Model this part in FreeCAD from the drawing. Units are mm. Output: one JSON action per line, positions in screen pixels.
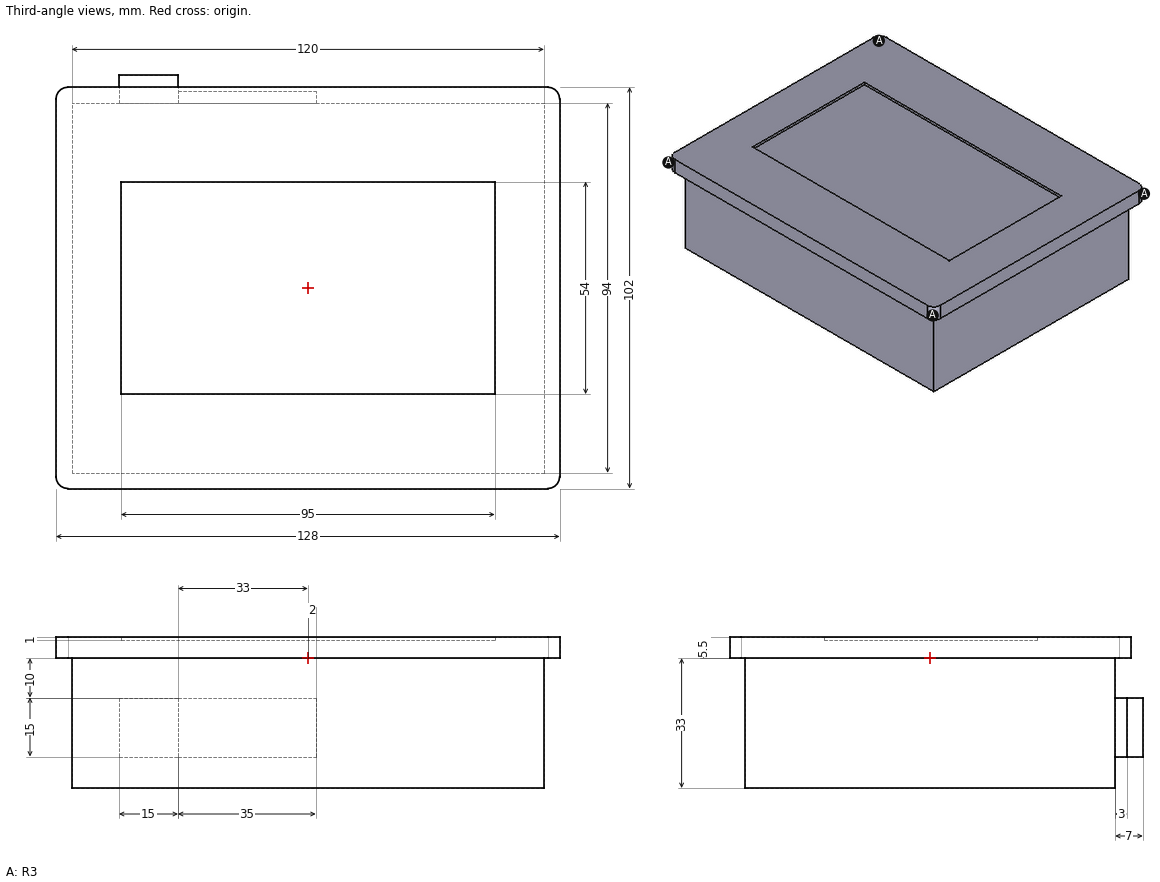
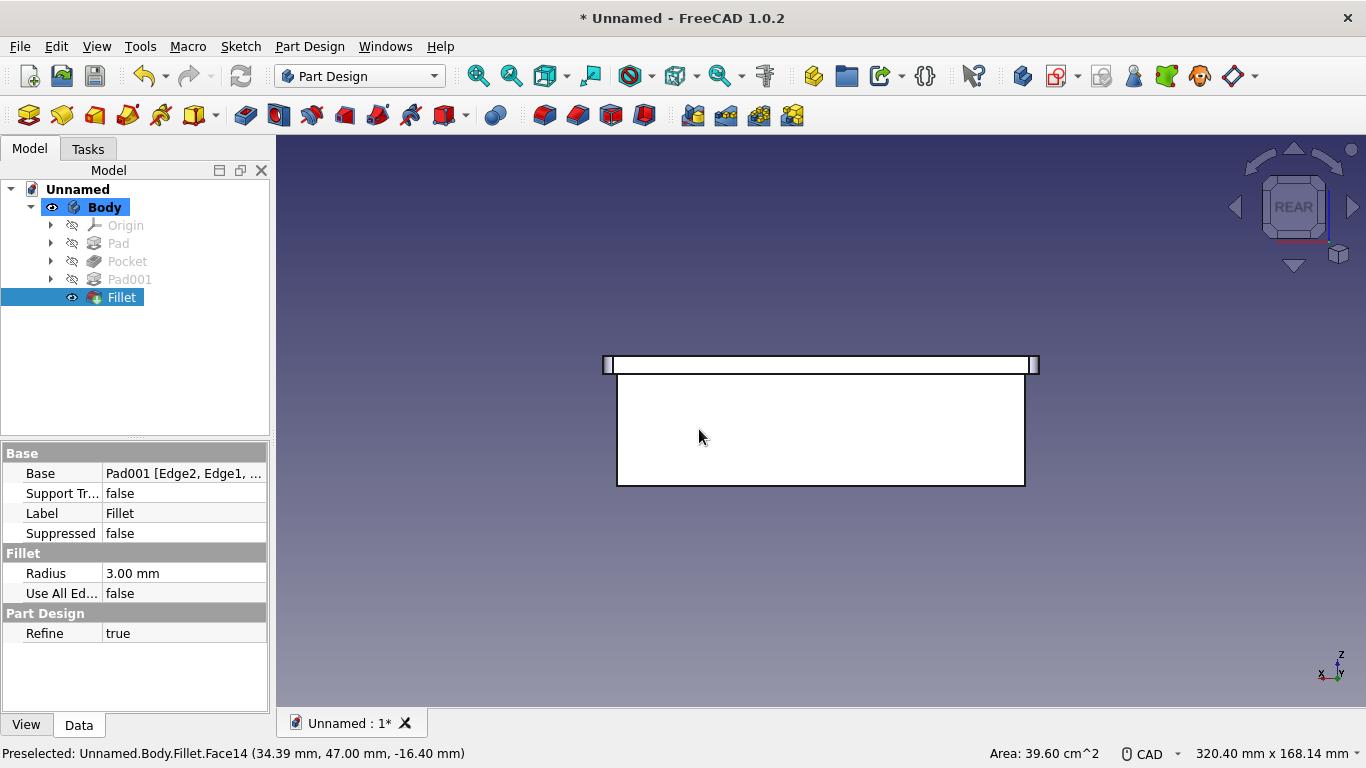
{"action": "left_click", "coordinate": [1056, 76]}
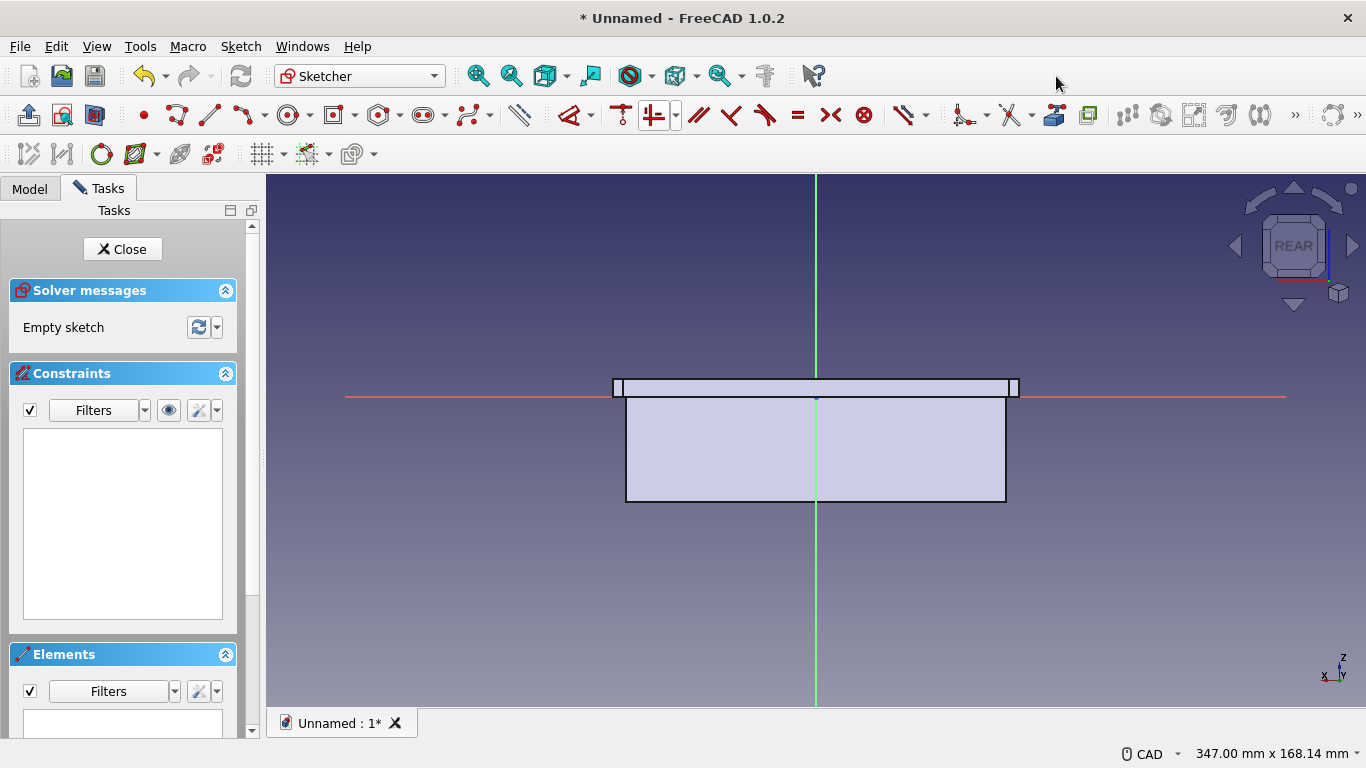
{"action": "key", "text": "q s"}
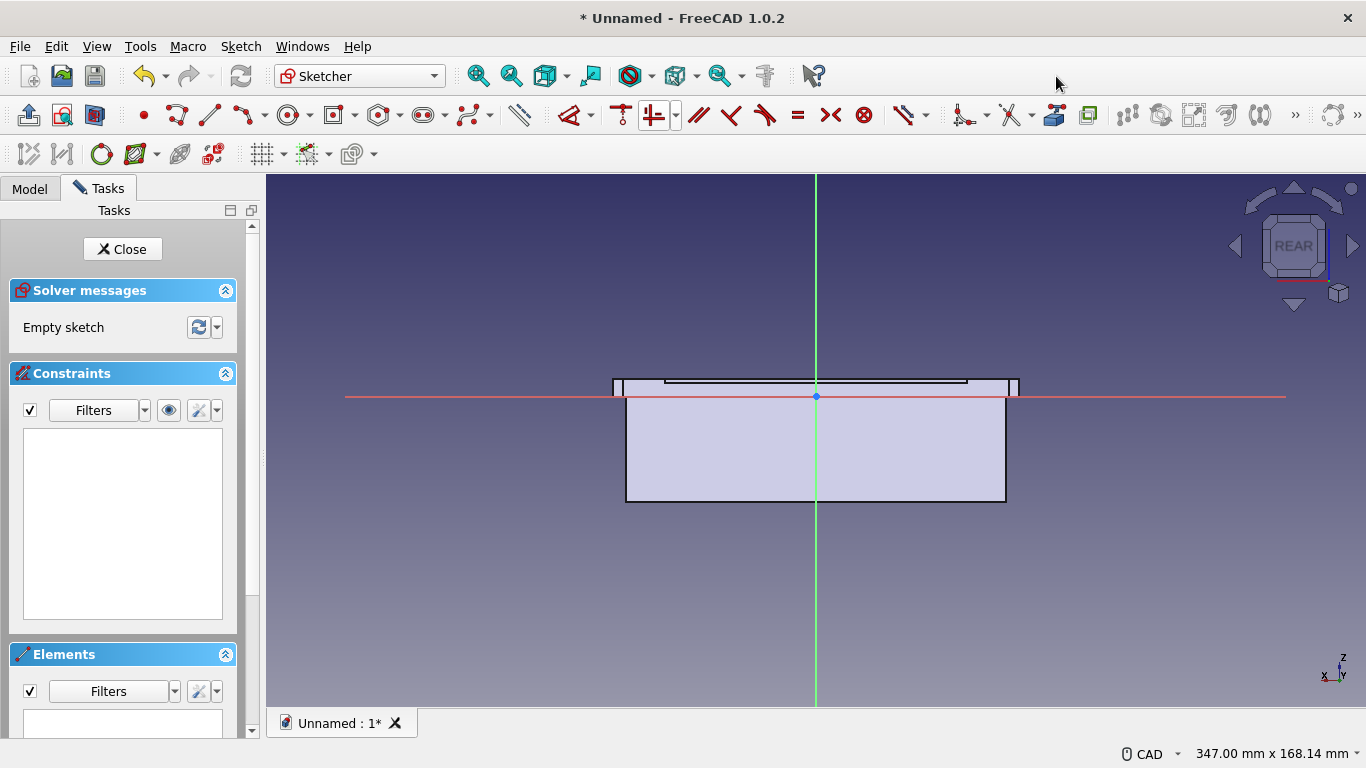
{"action": "scroll", "coordinate": [975, 454], "scroll_direction": "up", "scroll_amount": 10}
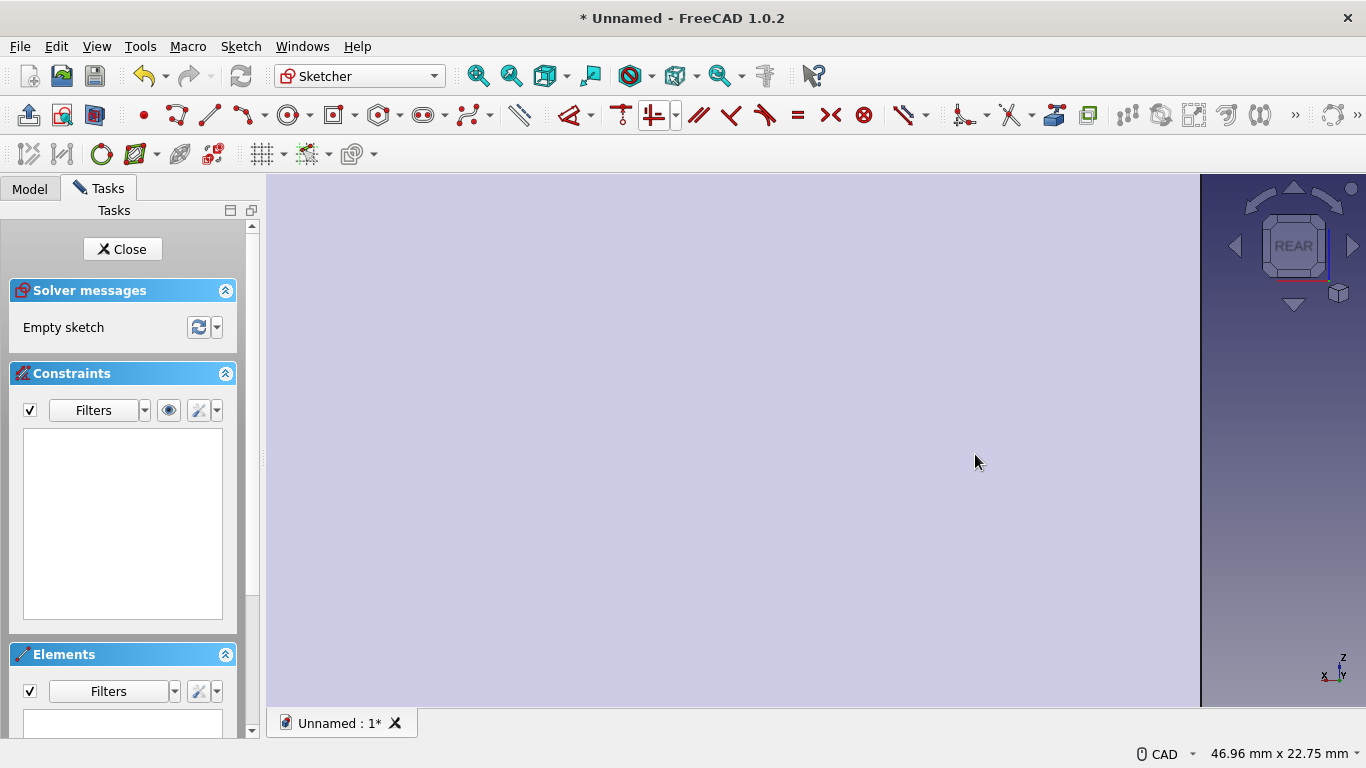
{"action": "key", "text": "g r"}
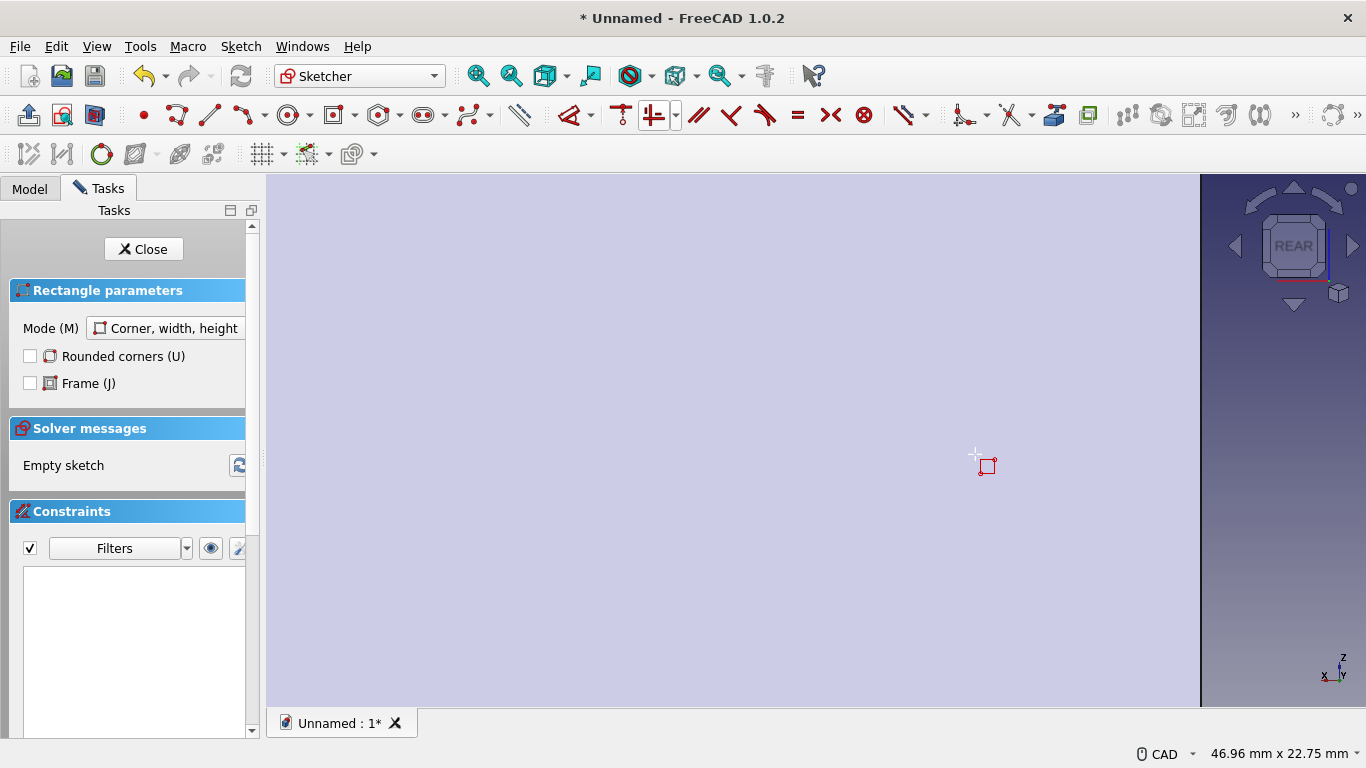
{"action": "left_click", "coordinate": [569, 263]}
{"action": "mouse_move", "coordinate": [920, 614]}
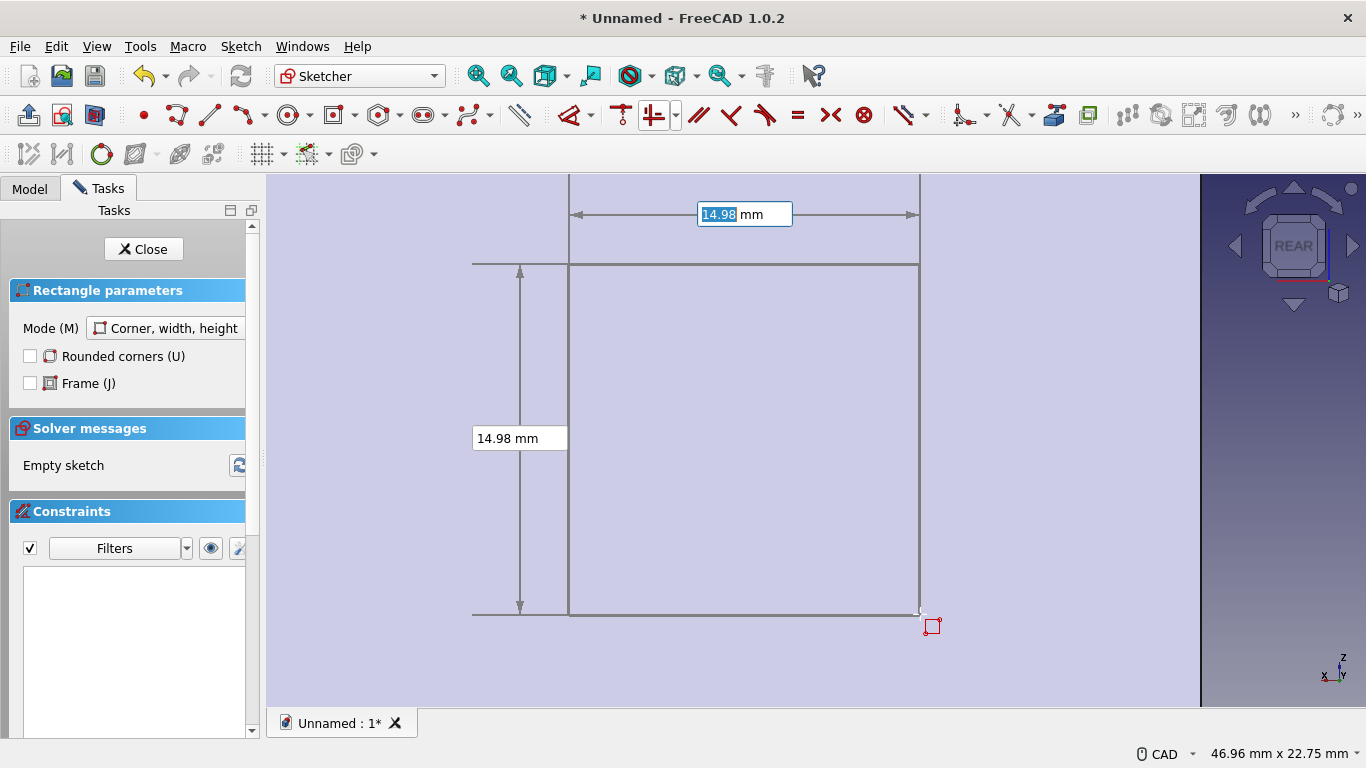
{"action": "type", "text": "15"}
{"action": "key", "text": "Tab"}
{"action": "type", "text": "15"}
{"action": "key", "text": "Return"}
{"action": "key", "text": "Escape"}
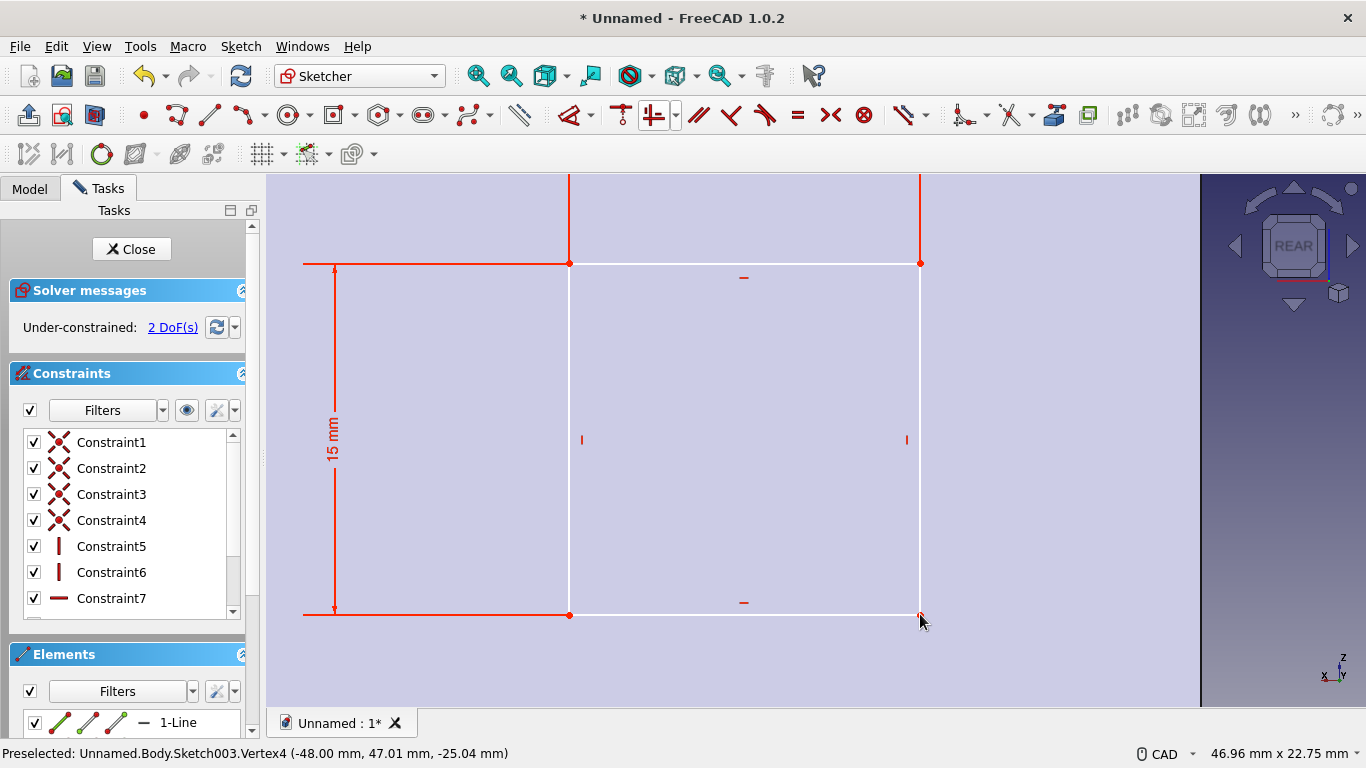
{"action": "left_click", "coordinate": [568, 116]}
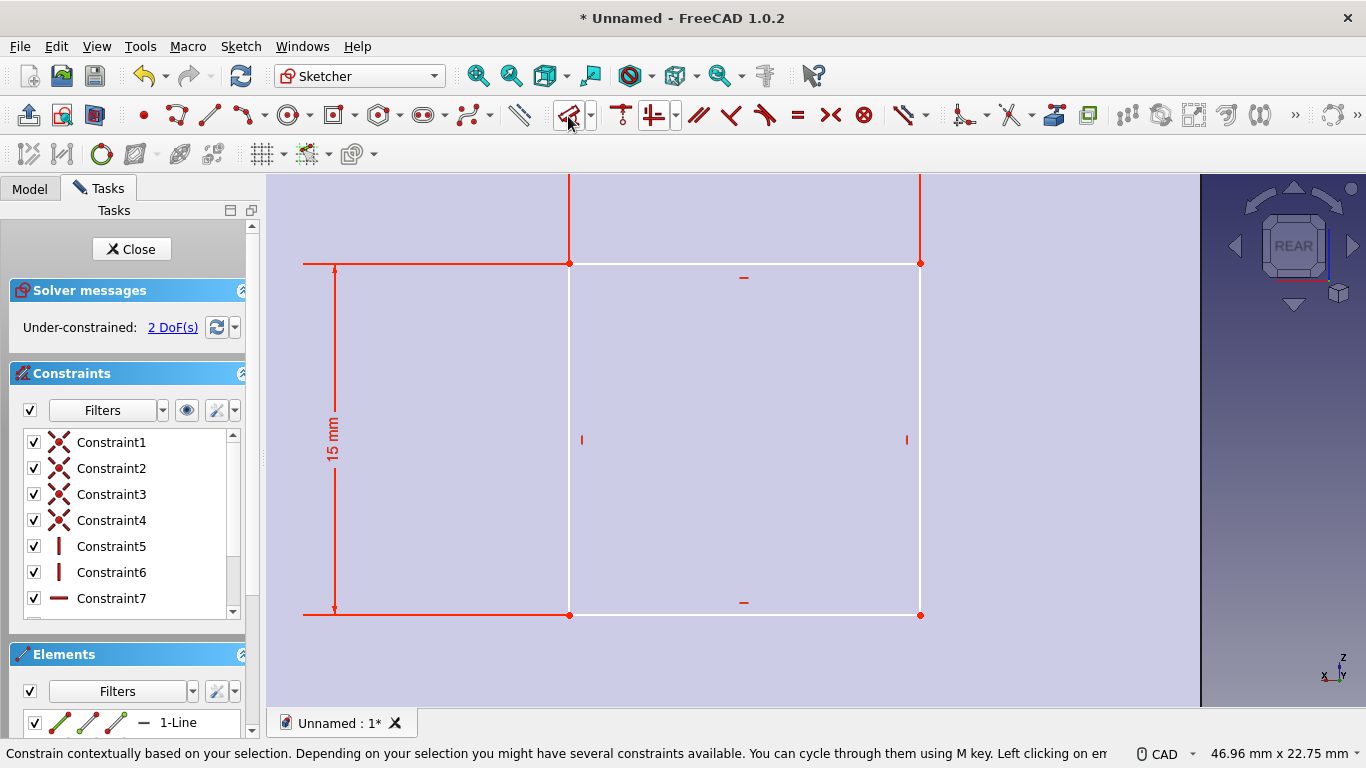
{"action": "left_click", "coordinate": [569, 264]}
{"action": "left_click", "coordinate": [431, 298]}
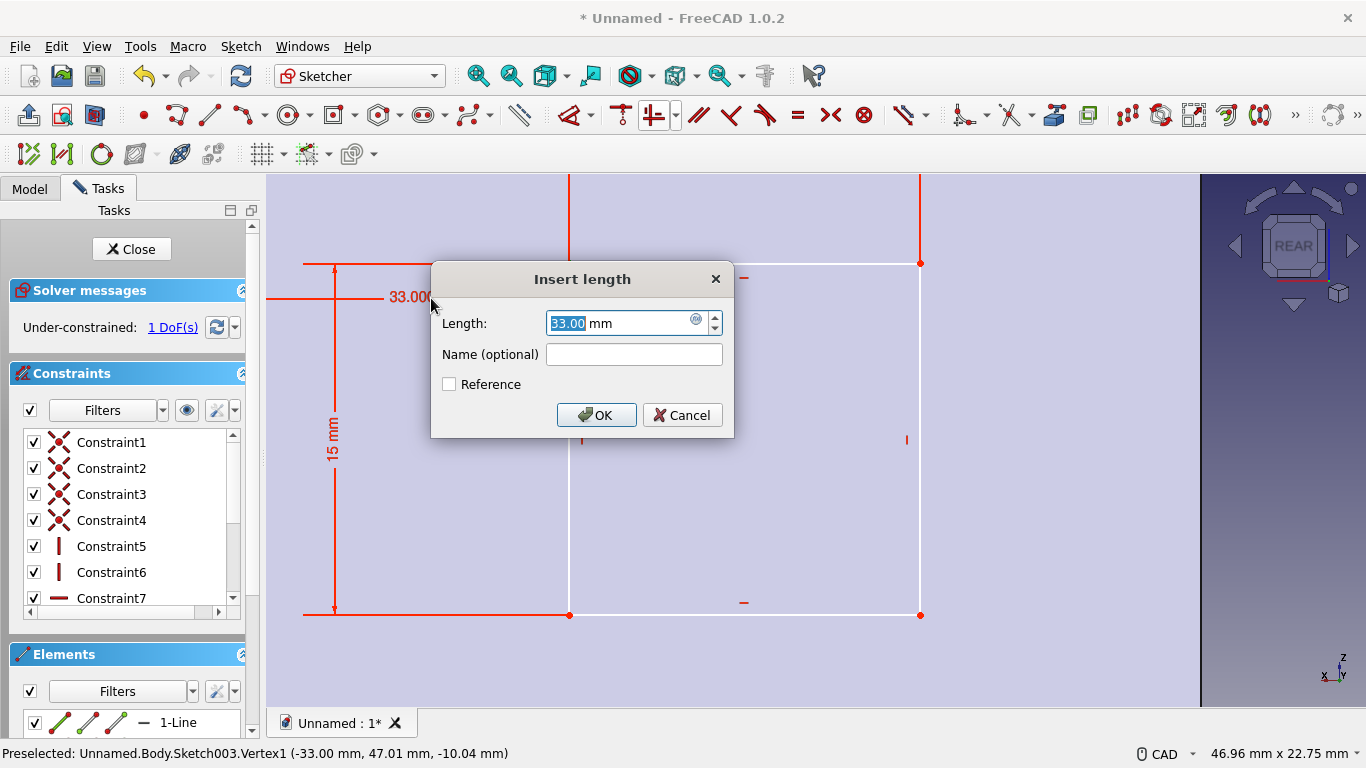
{"action": "type", "text": "33"}
{"action": "key", "text": "Return"}